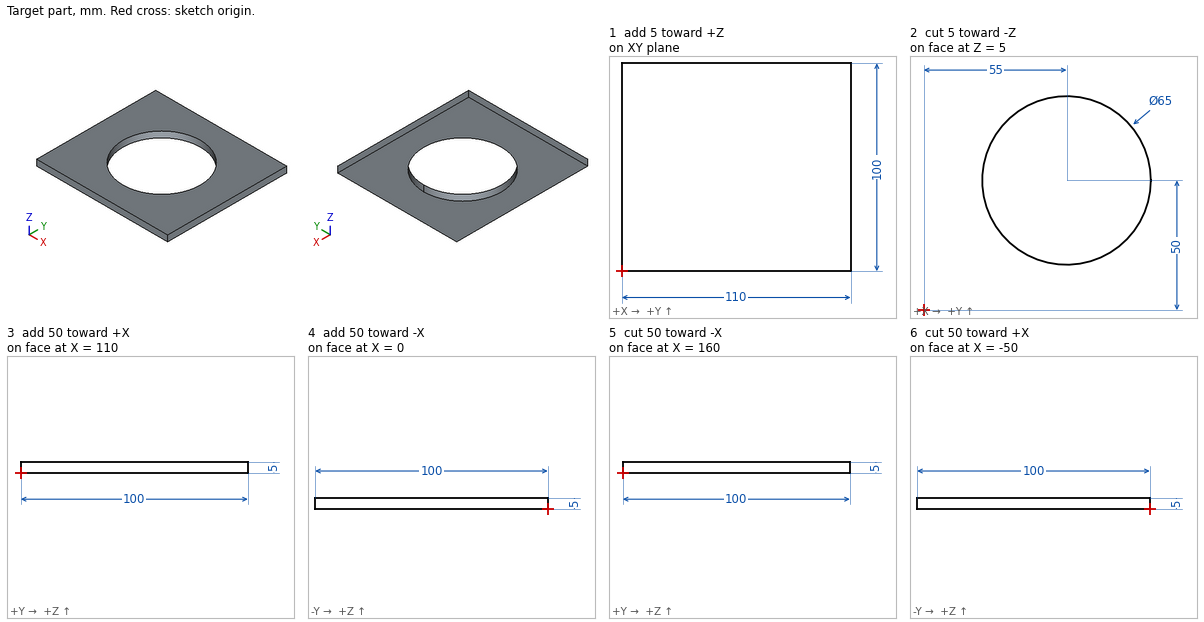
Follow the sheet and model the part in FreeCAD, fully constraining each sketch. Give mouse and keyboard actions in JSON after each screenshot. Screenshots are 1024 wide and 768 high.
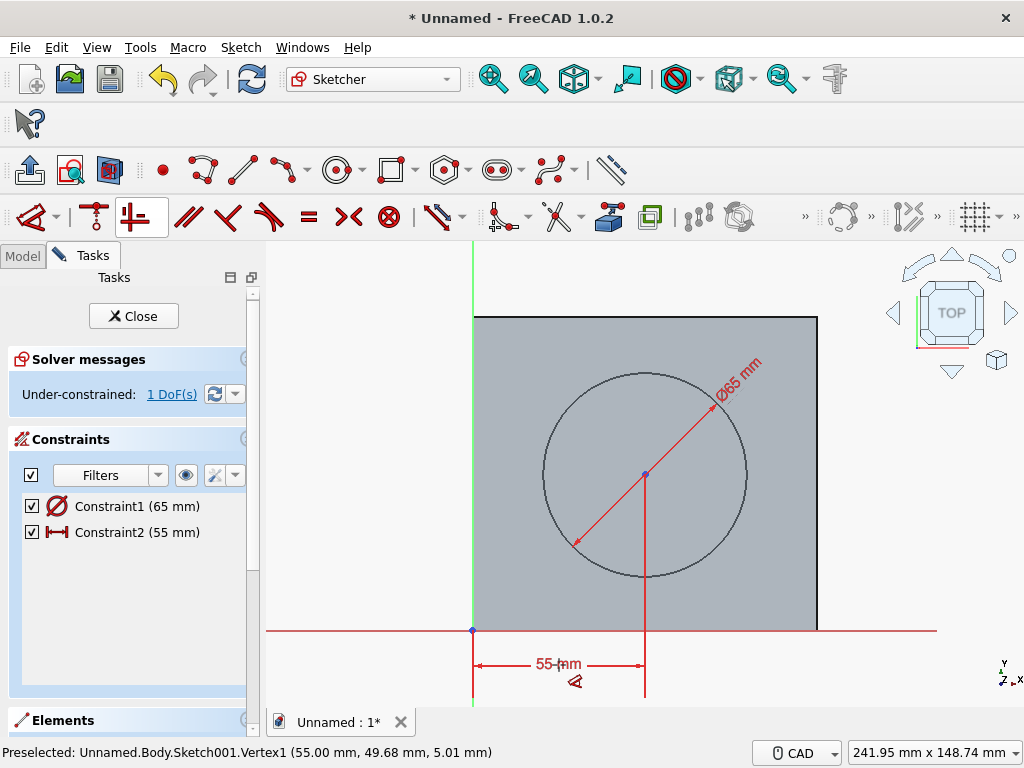
{"action": "left_click", "coordinate": [645, 475]}
{"action": "left_click", "coordinate": [439, 553]}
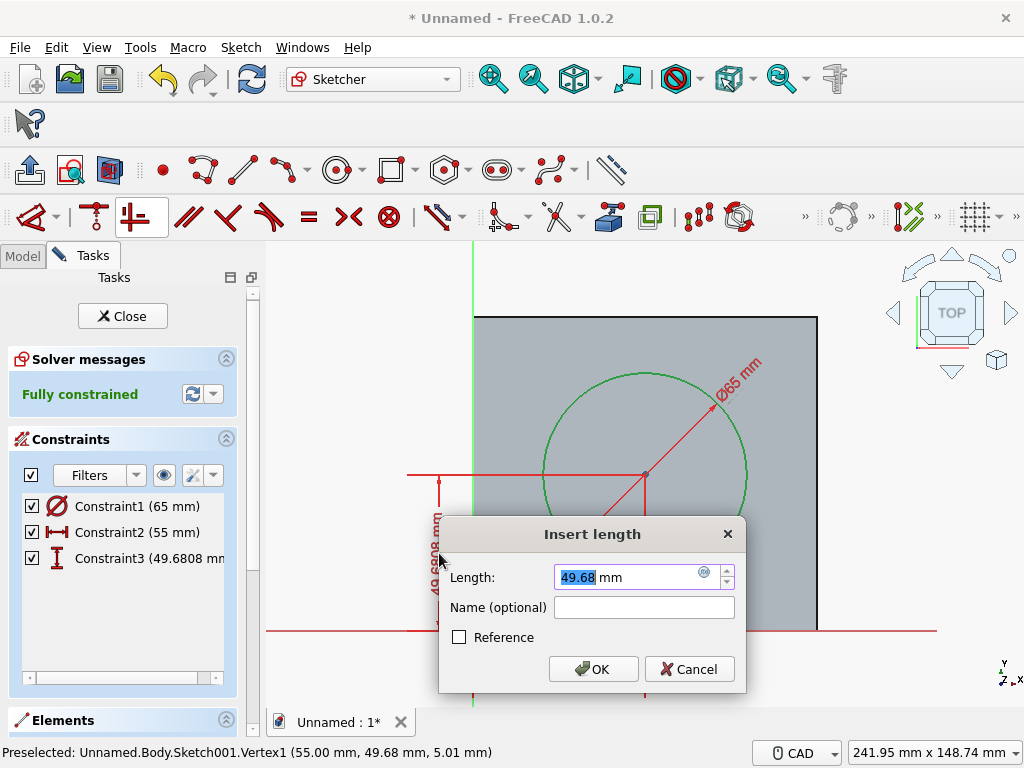
{"action": "type", "text": "50"}
{"action": "key", "text": "Return"}
{"action": "key", "text": "Escape"}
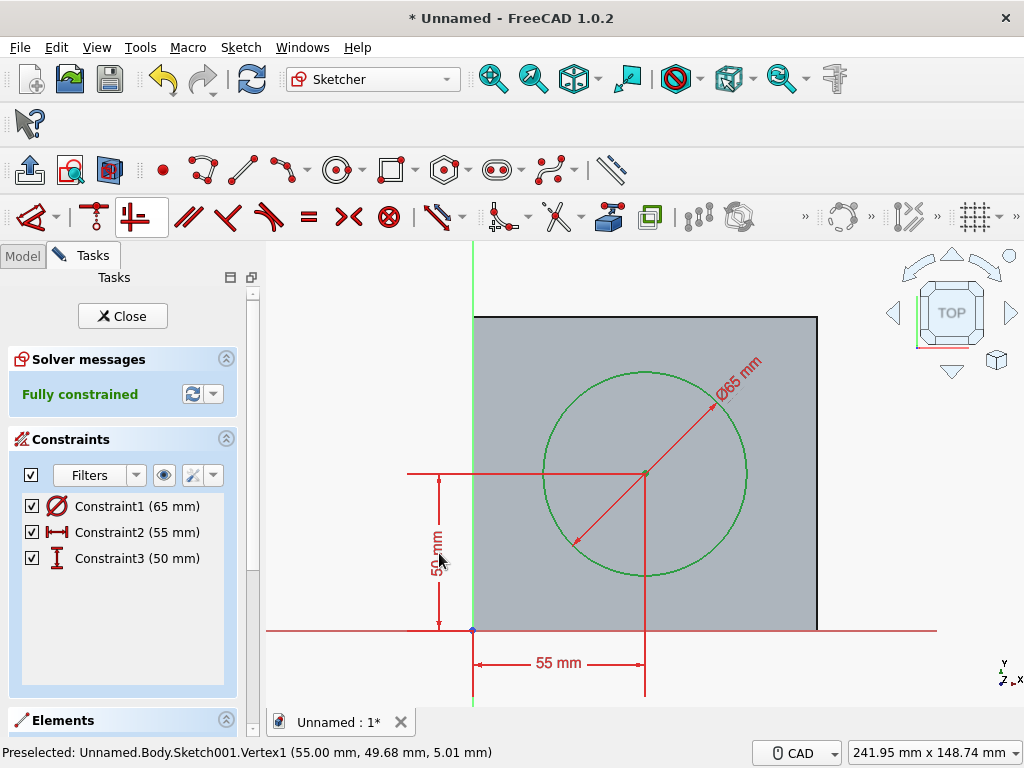
{"action": "left_click", "coordinate": [123, 316]}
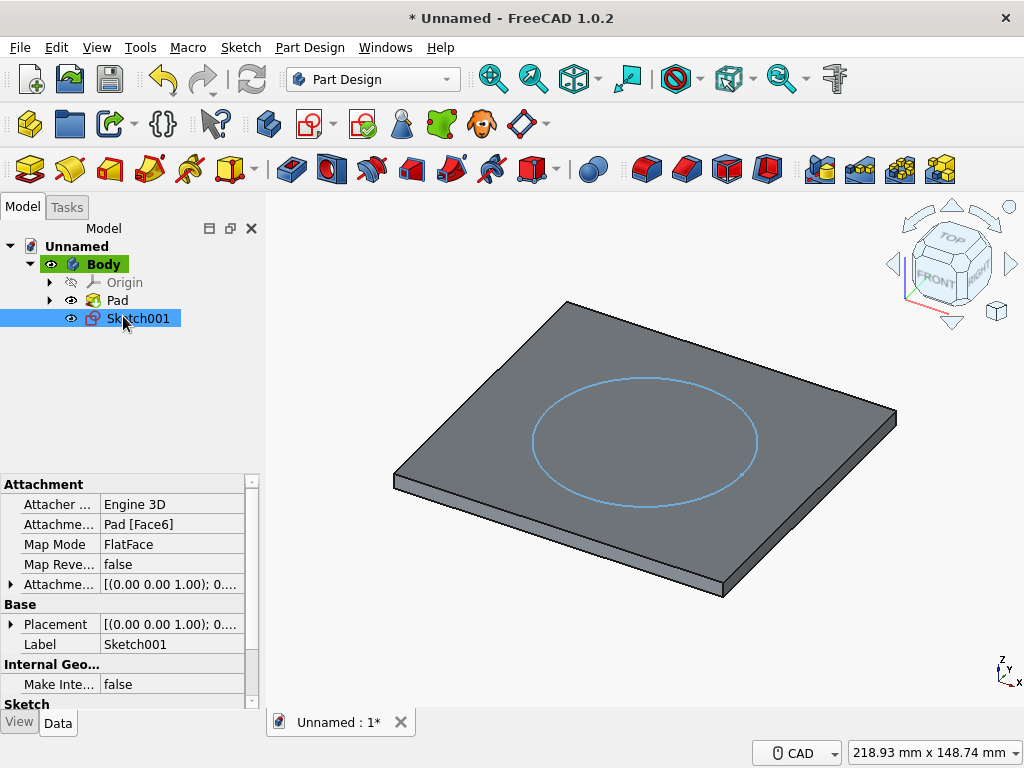
{"action": "left_click", "coordinate": [292, 170]}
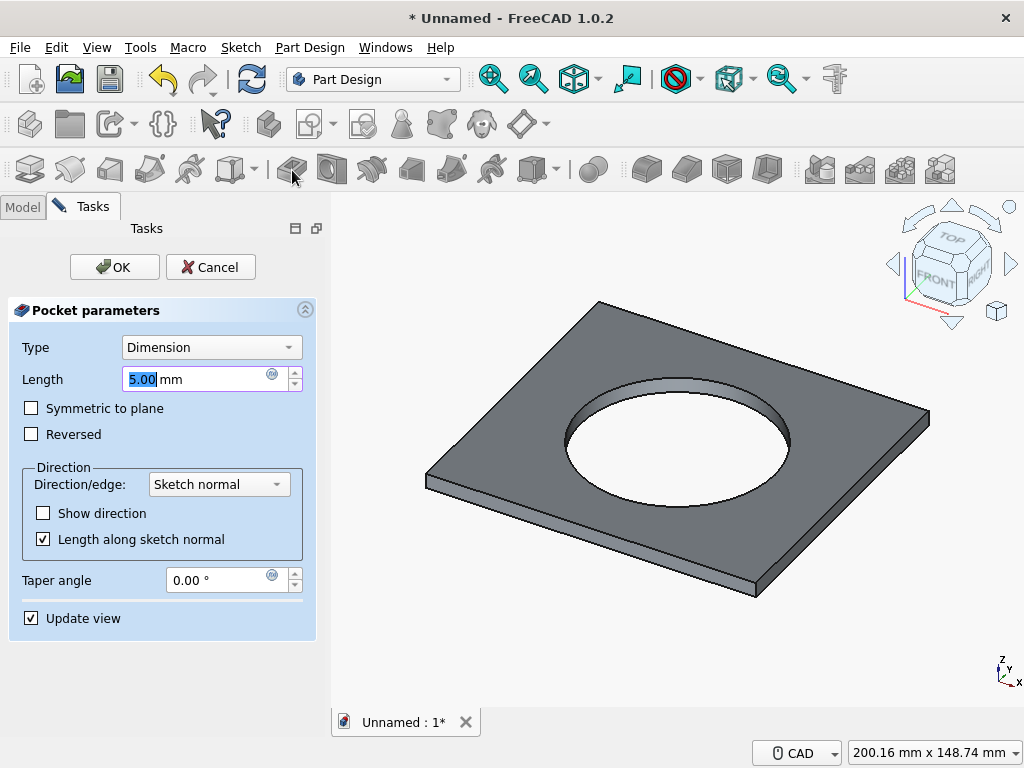
{"action": "type", "text": "5"}
{"action": "key", "text": "Tab"}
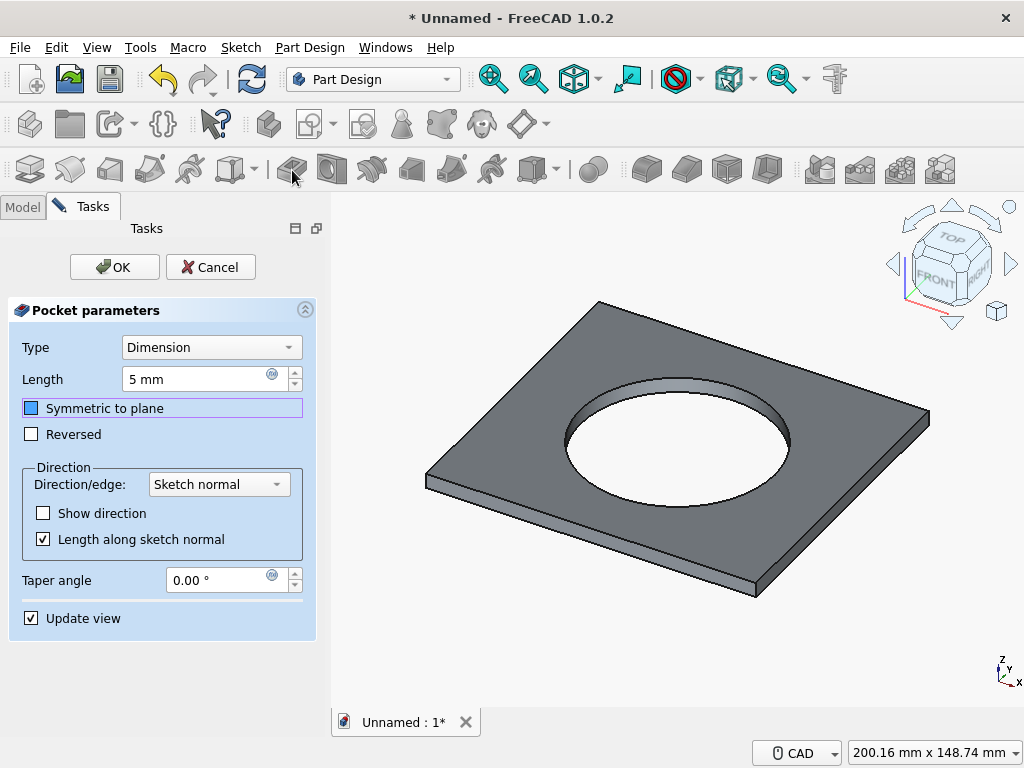
{"action": "left_click", "coordinate": [115, 267]}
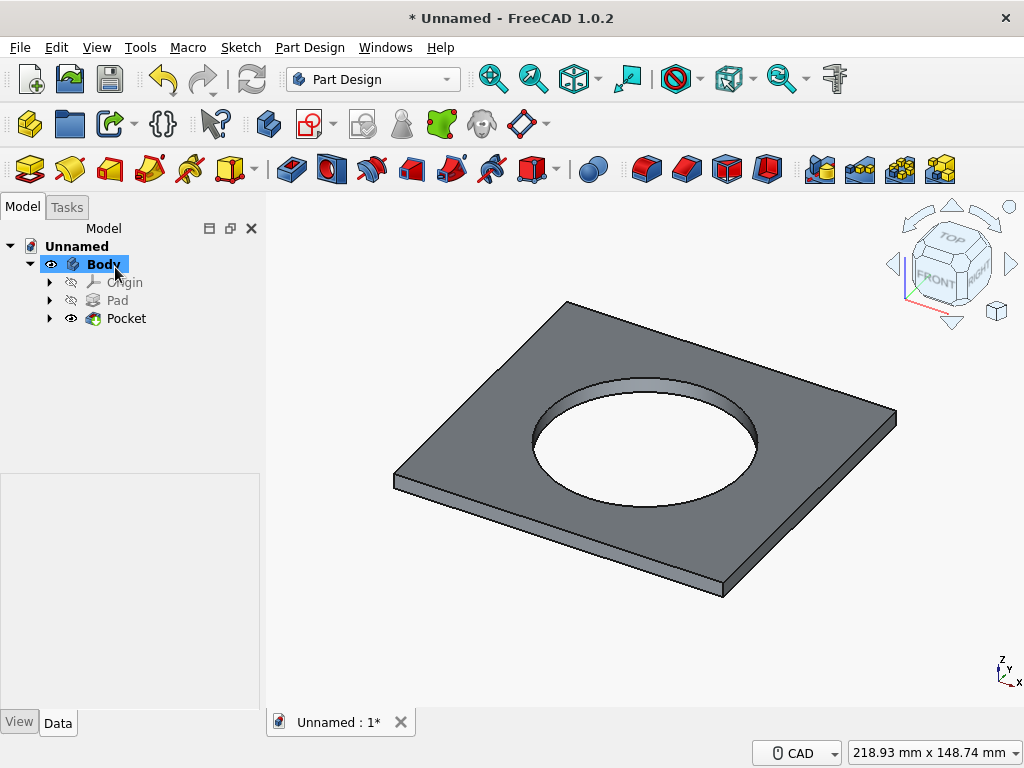
{"action": "key", "text": "0"}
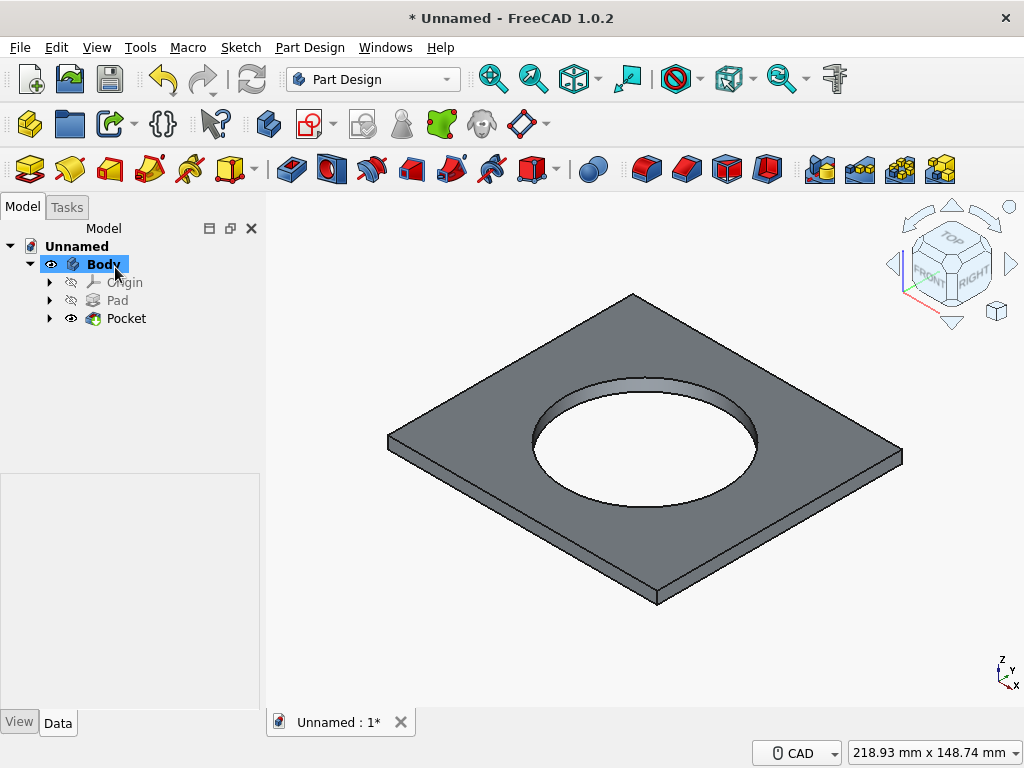
{"action": "key", "text": "3"}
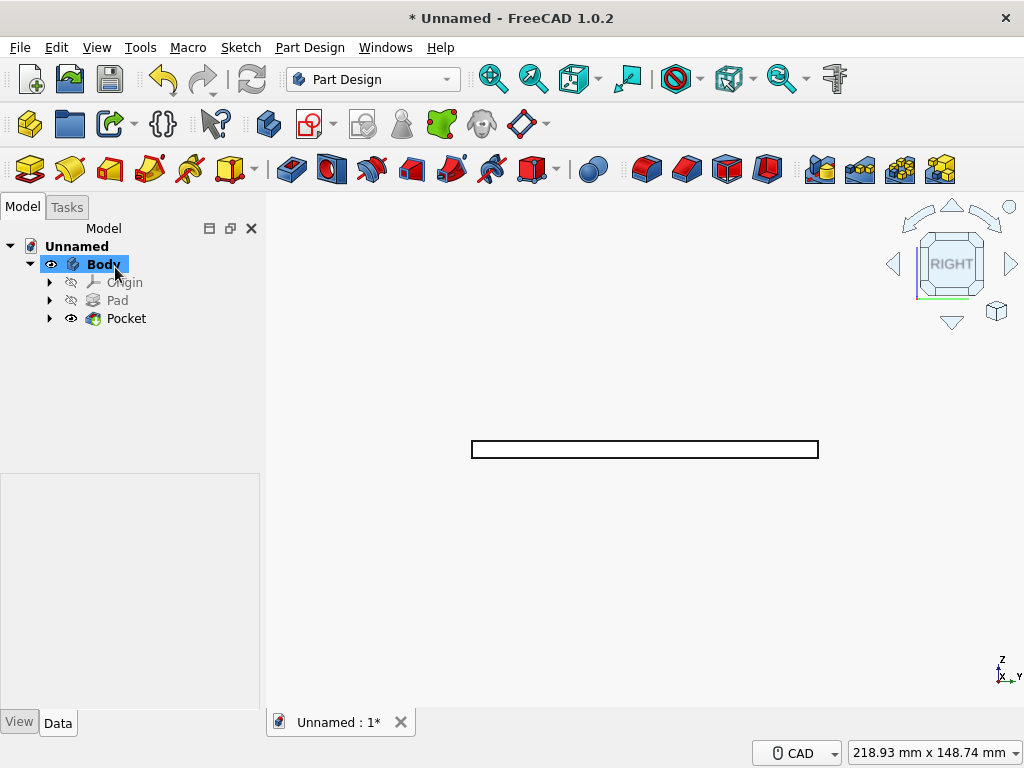
{"action": "left_click", "coordinate": [793, 448]}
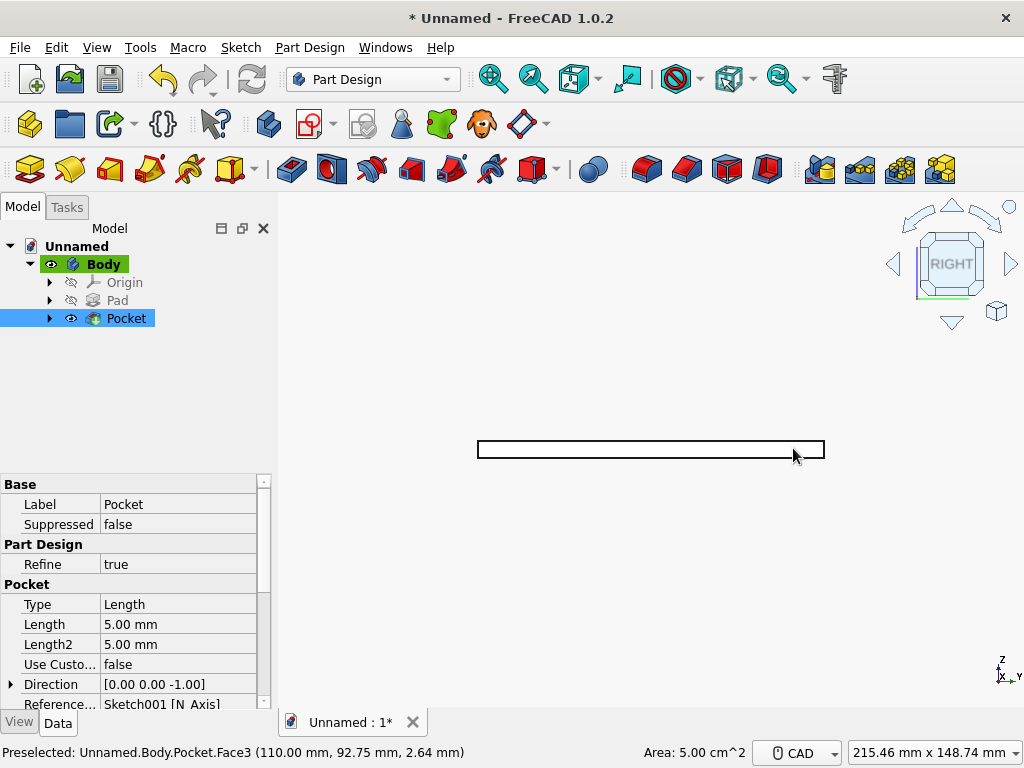
{"action": "left_click", "coordinate": [310, 124]}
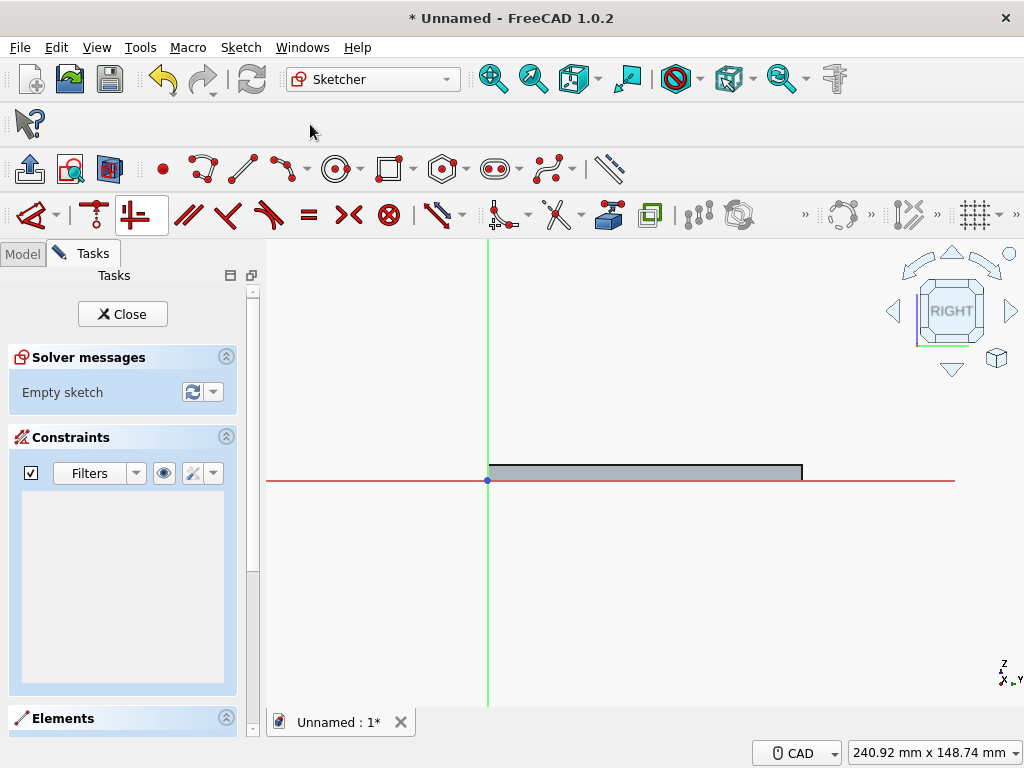
{"action": "left_click", "coordinate": [390, 170]}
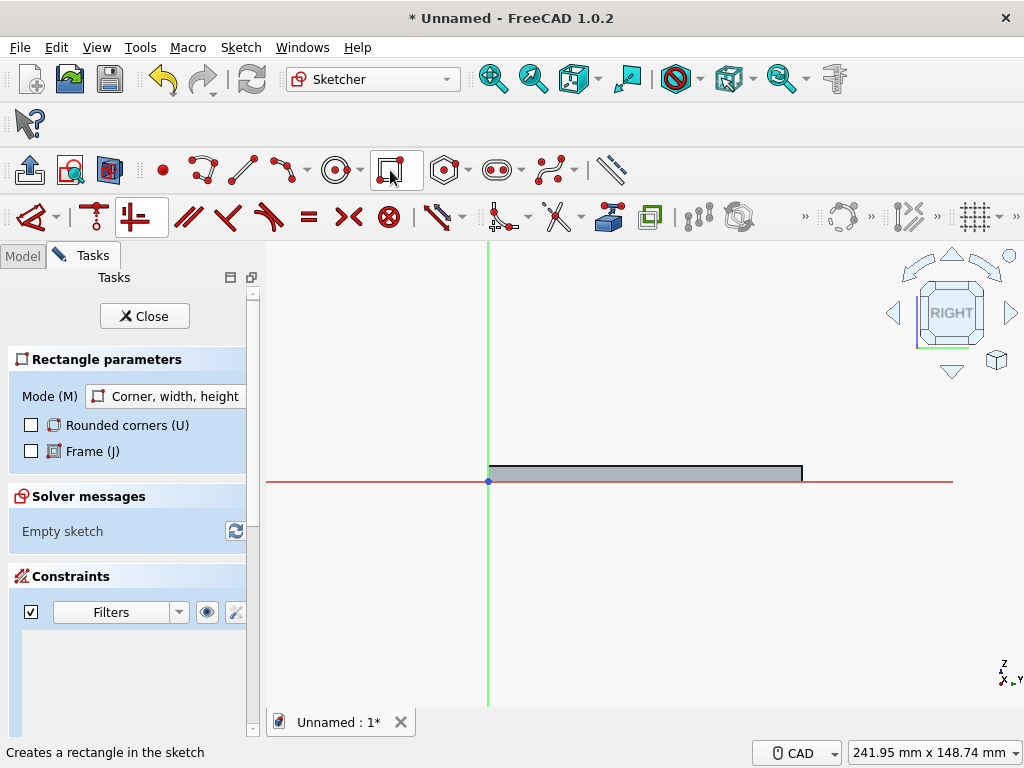
{"action": "left_click", "coordinate": [488, 482]}
{"action": "left_click", "coordinate": [802, 466]}
{"action": "key", "text": "Escape"}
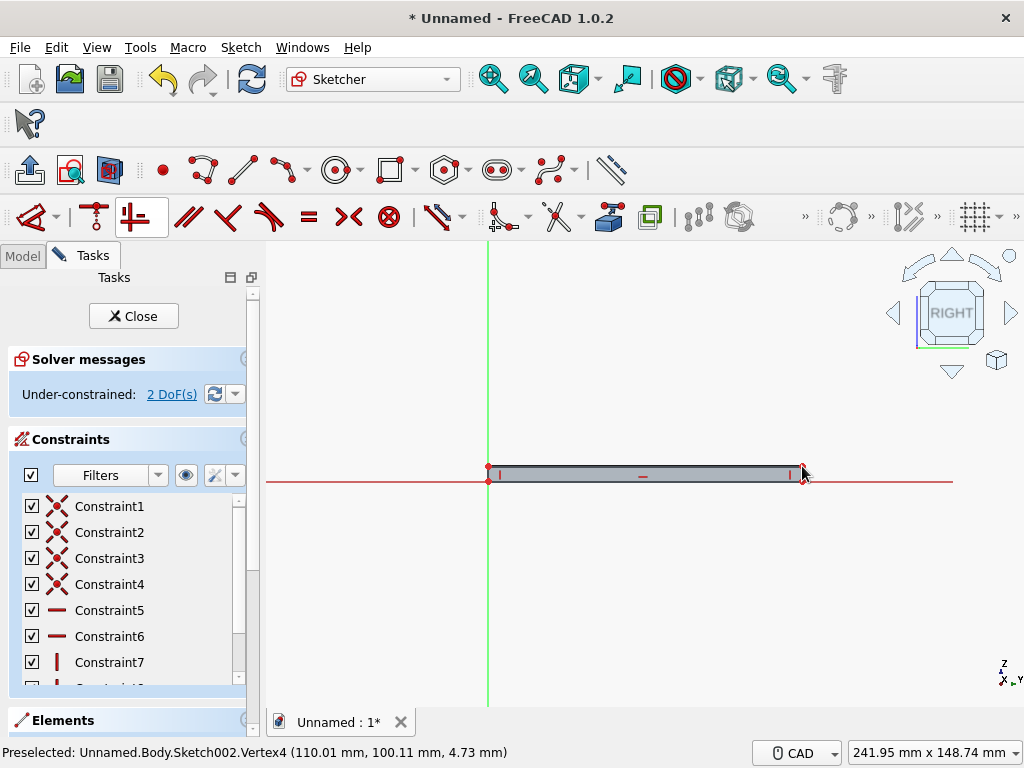
{"action": "left_click", "coordinate": [32, 218]}